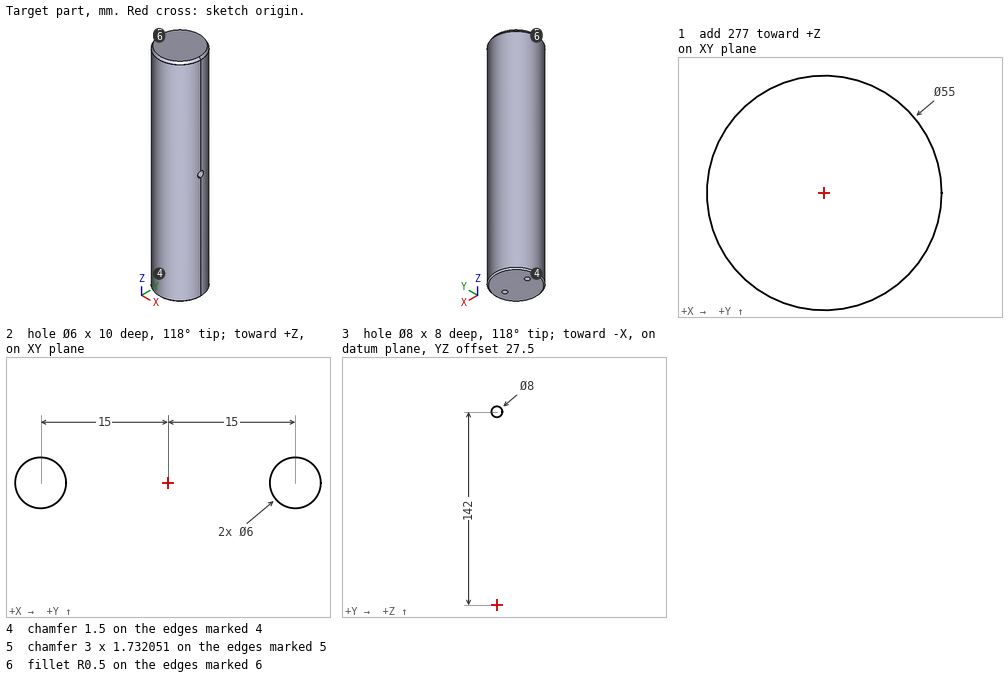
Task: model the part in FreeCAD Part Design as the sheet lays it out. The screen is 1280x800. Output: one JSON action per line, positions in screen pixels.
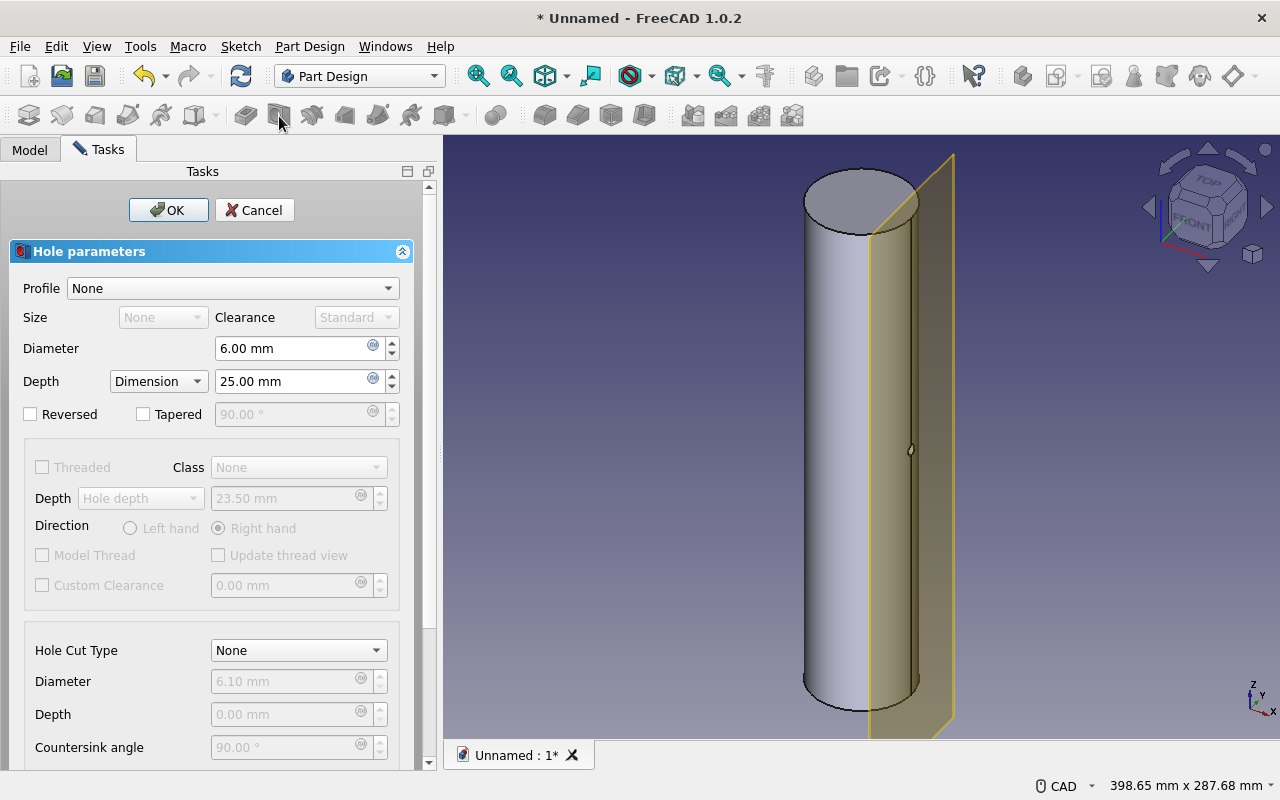
{"action": "triple_click", "coordinate": [300, 348]}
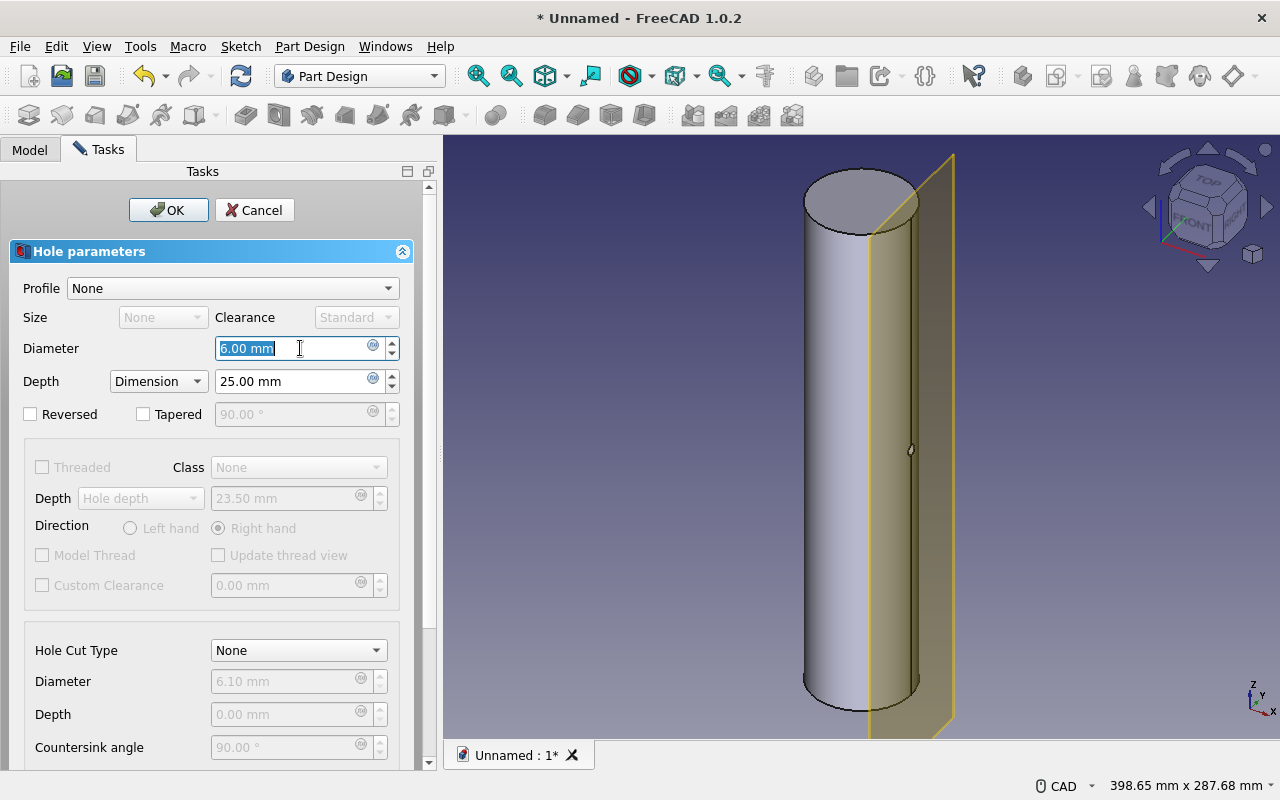
{"action": "type", "text": "8"}
{"action": "key", "text": "Tab"}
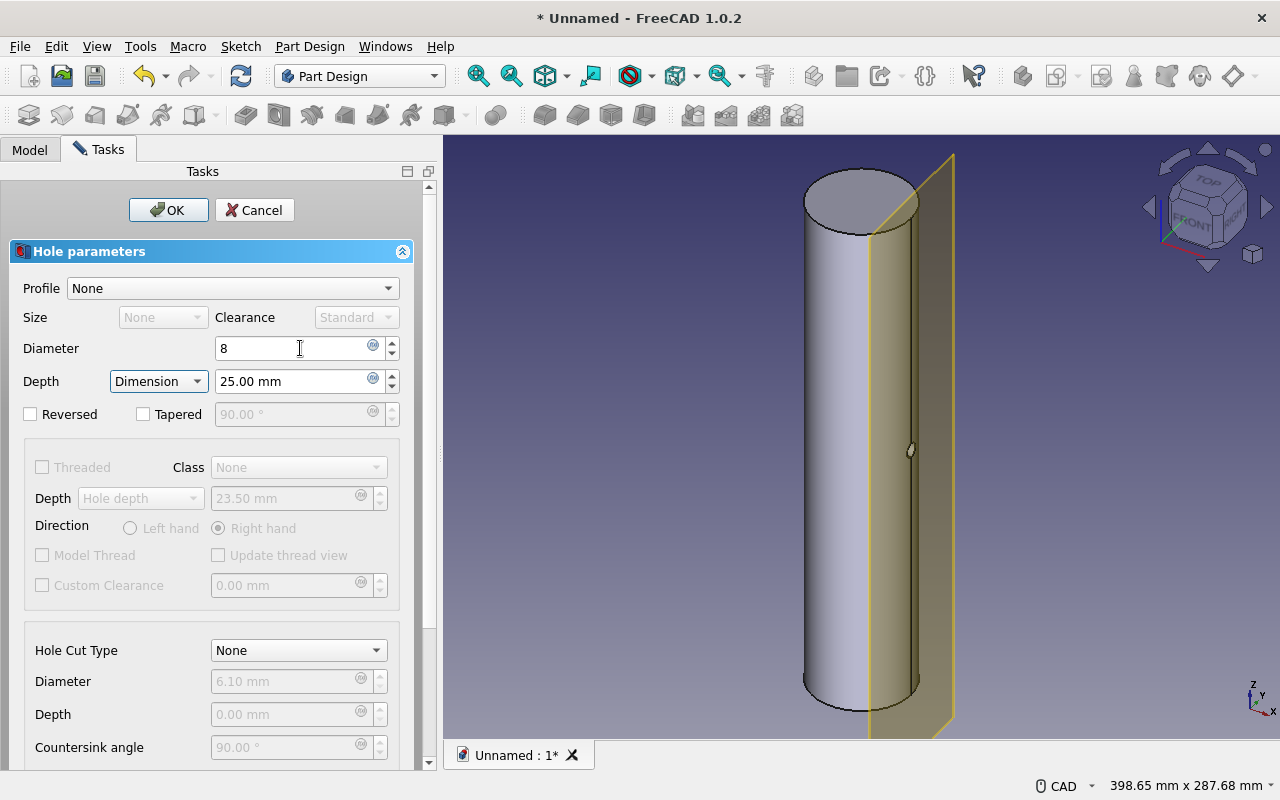
{"action": "triple_click", "coordinate": [300, 382]}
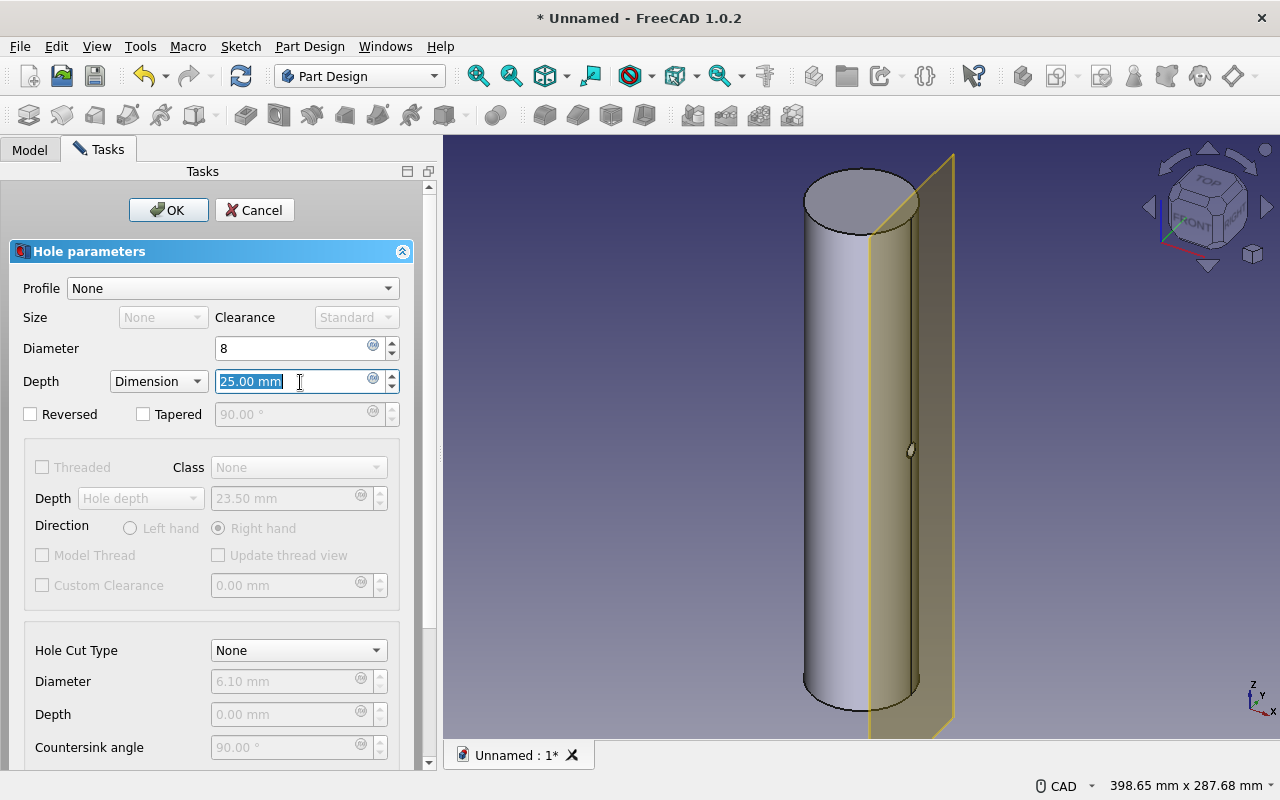
{"action": "type", "text": "8"}
{"action": "key", "text": "Tab"}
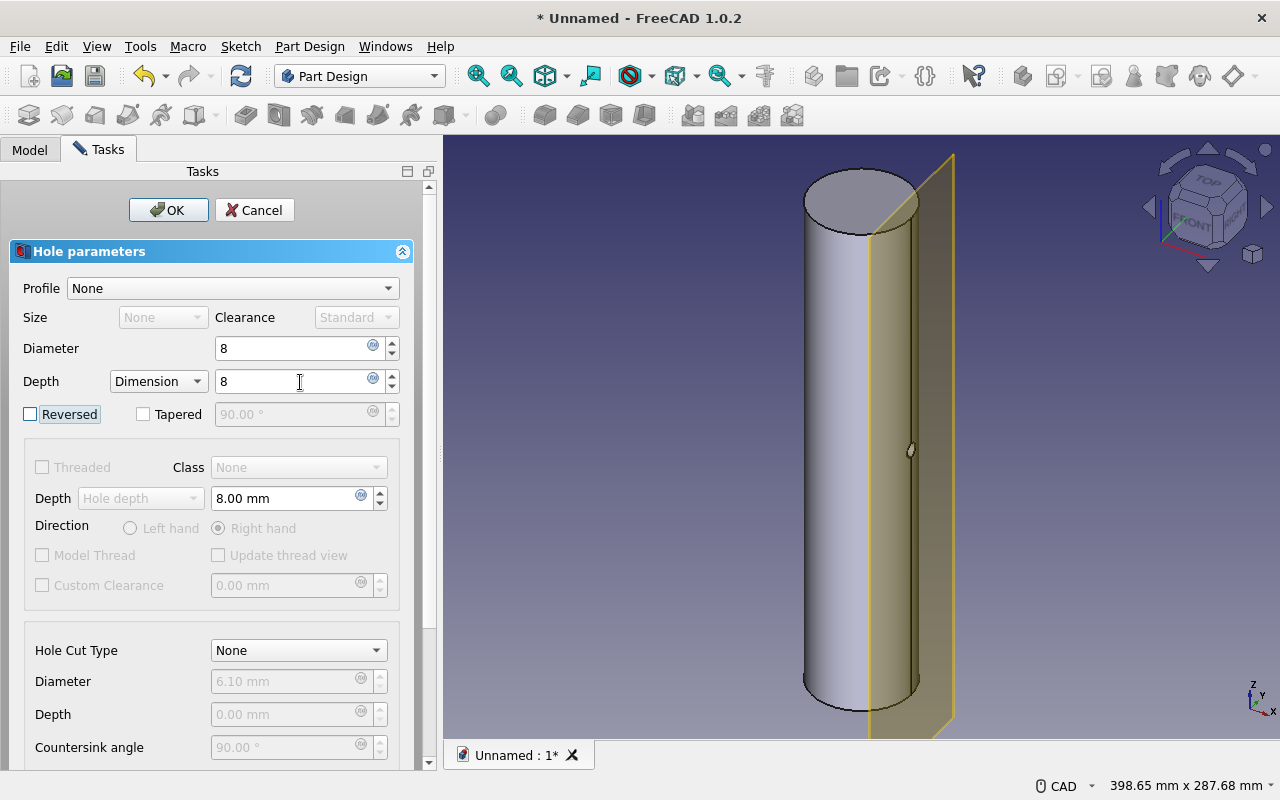
{"action": "left_click", "coordinate": [169, 210]}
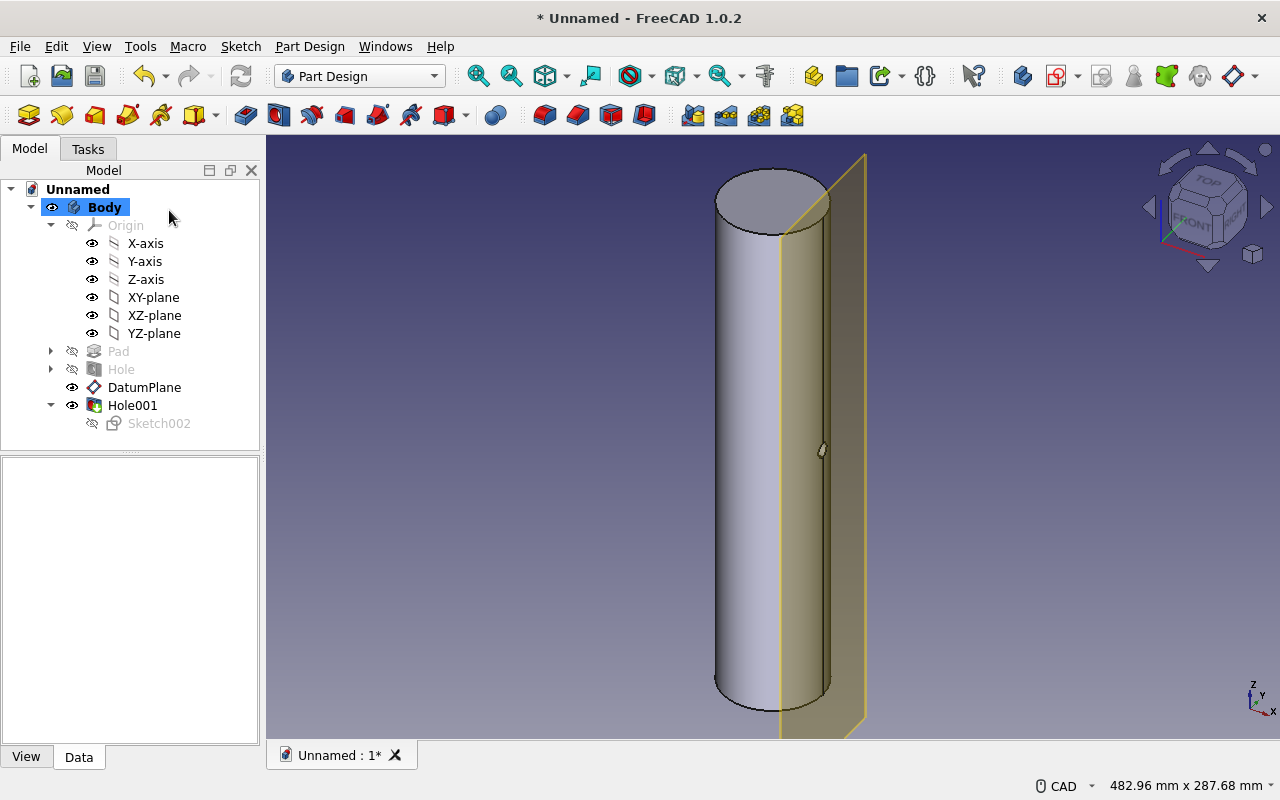
{"action": "left_click", "coordinate": [117, 387]}
{"action": "key", "text": "space"}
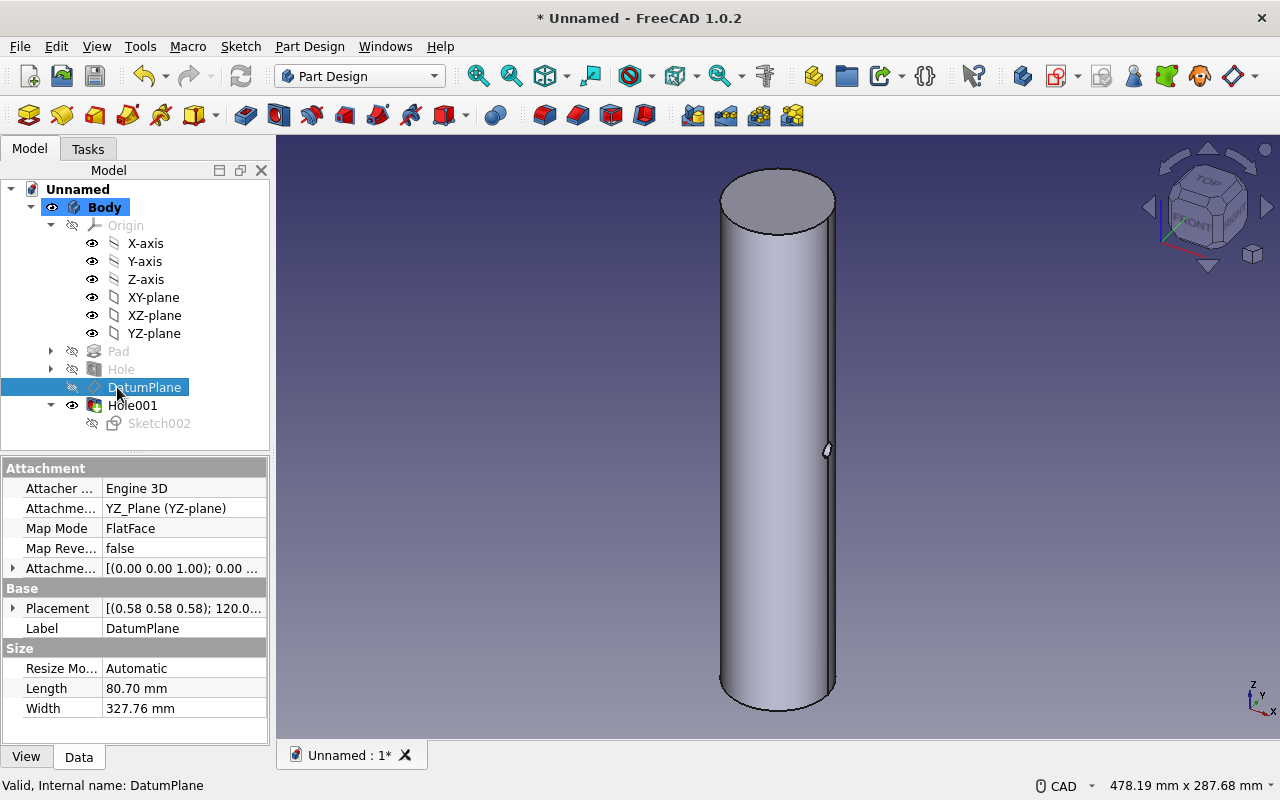
{"action": "key", "text": "0"}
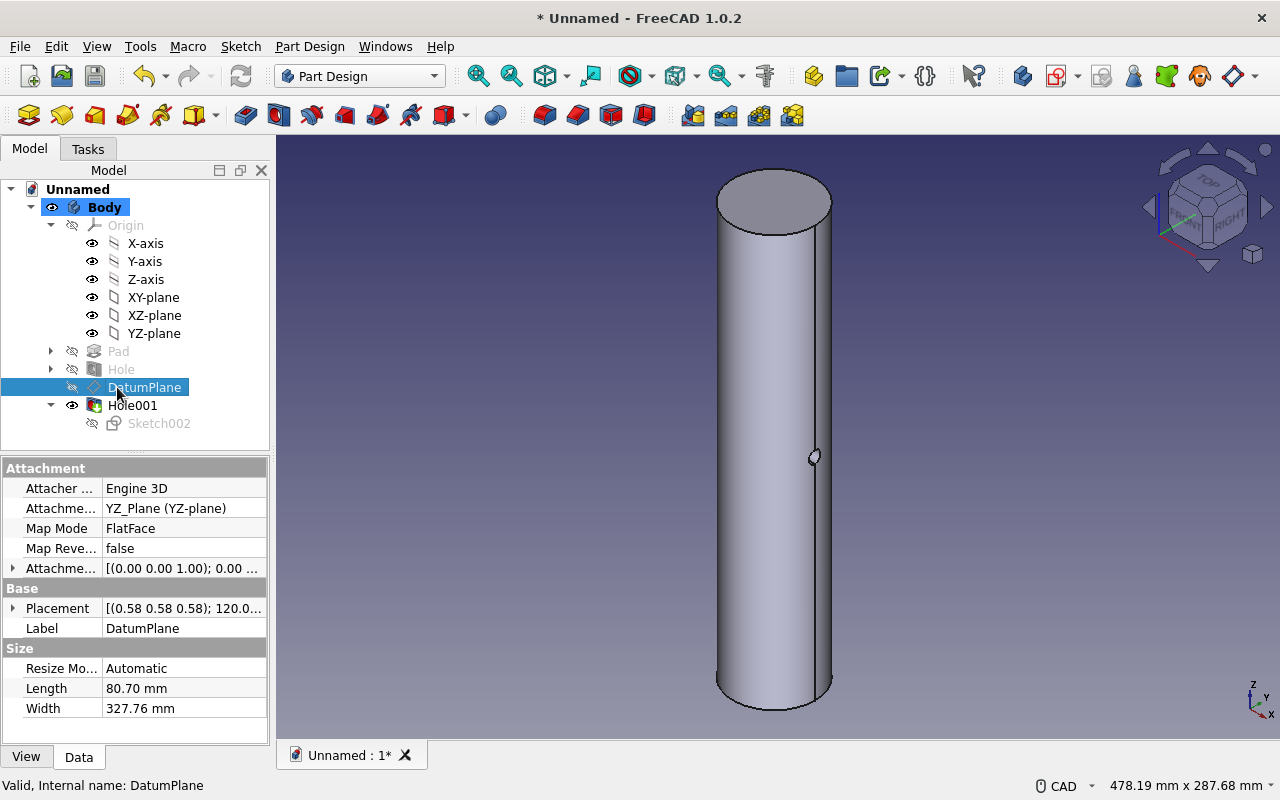
{"action": "key", "text": "2"}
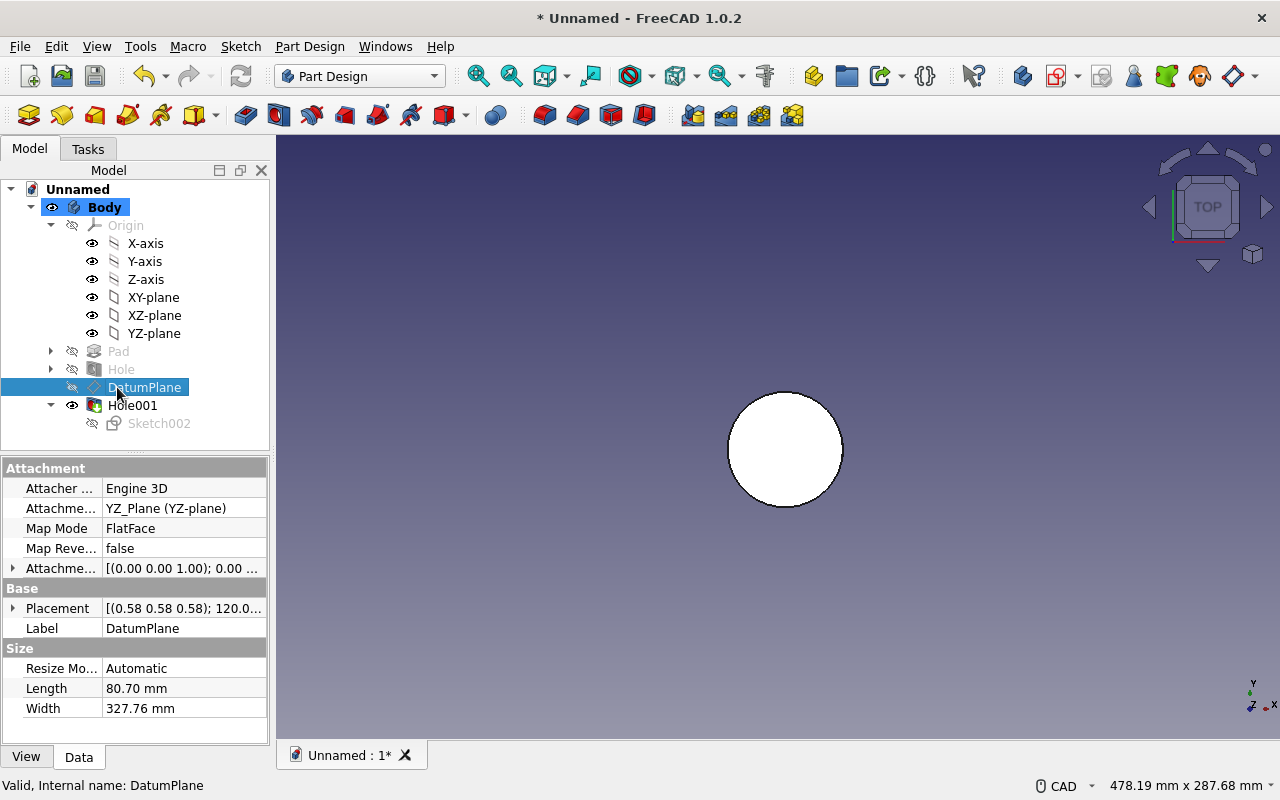
{"action": "key", "text": "v f"}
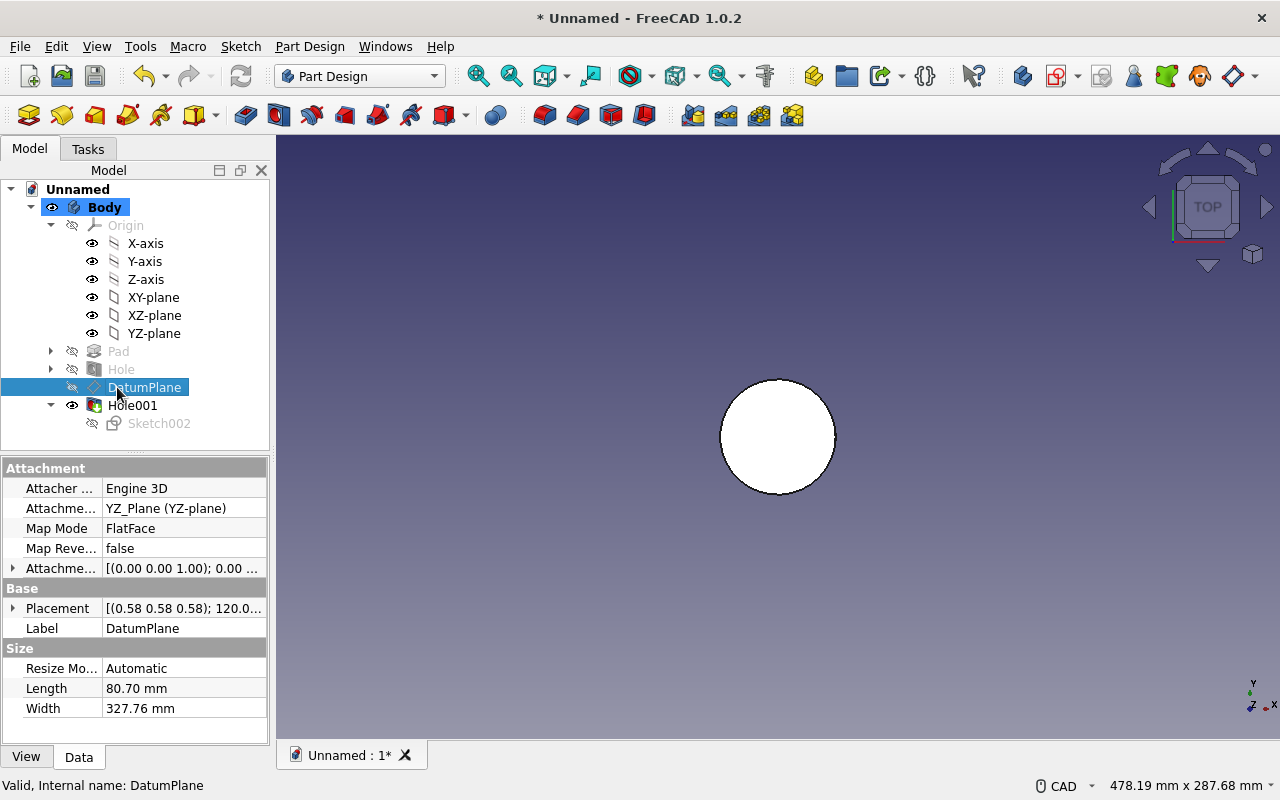
{"action": "key", "text": "1"}